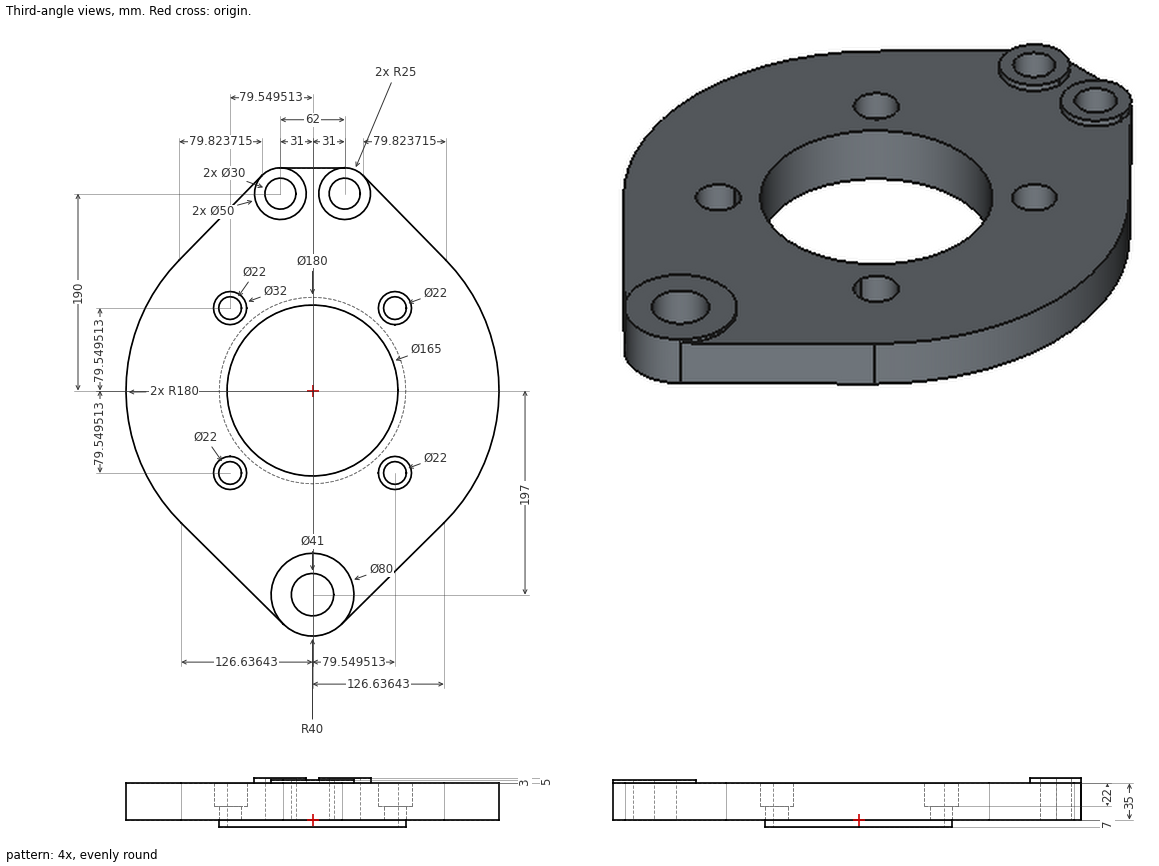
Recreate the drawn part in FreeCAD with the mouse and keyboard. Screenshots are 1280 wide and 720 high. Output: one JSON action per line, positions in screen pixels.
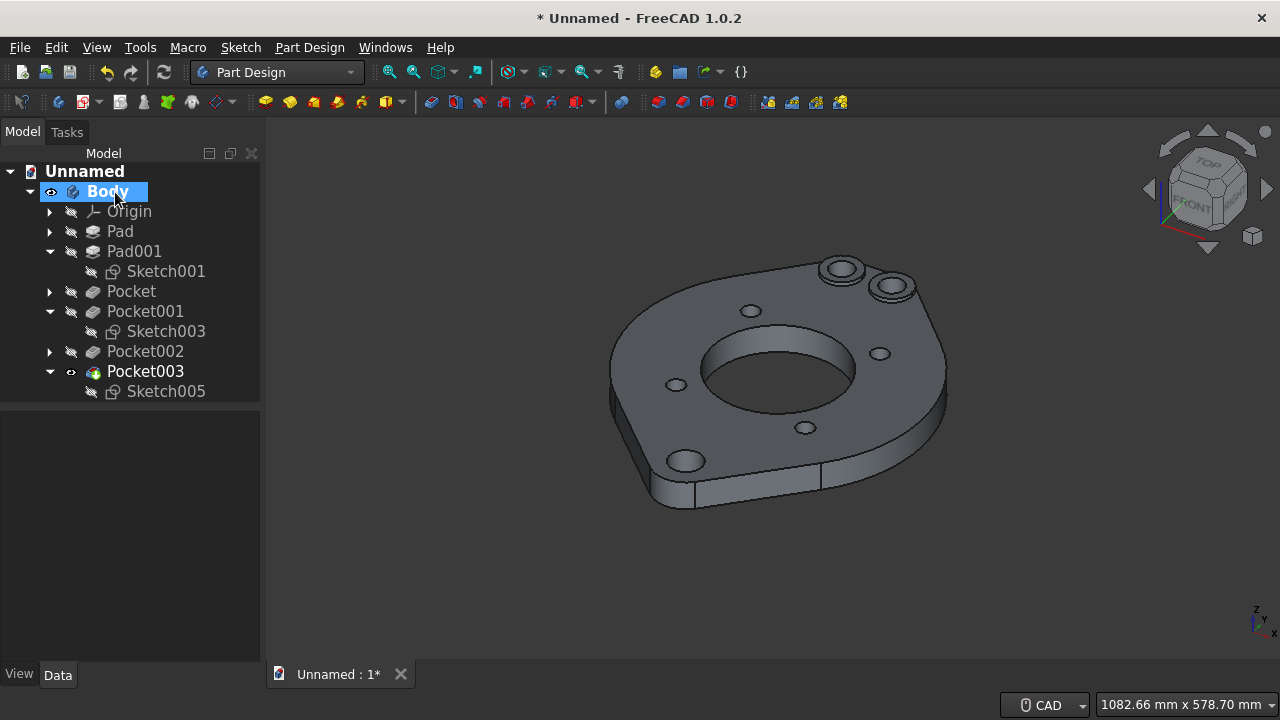
{"action": "left_click", "coordinate": [671, 420]}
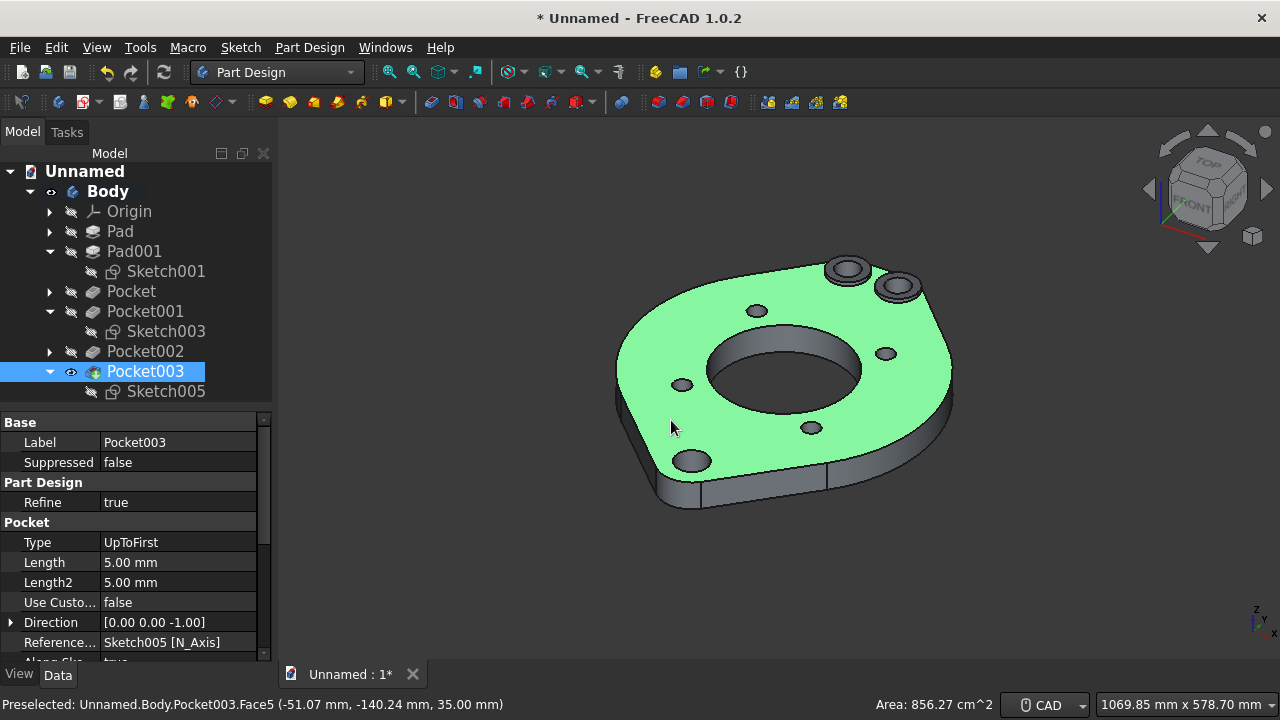
{"action": "left_click", "coordinate": [84, 102]}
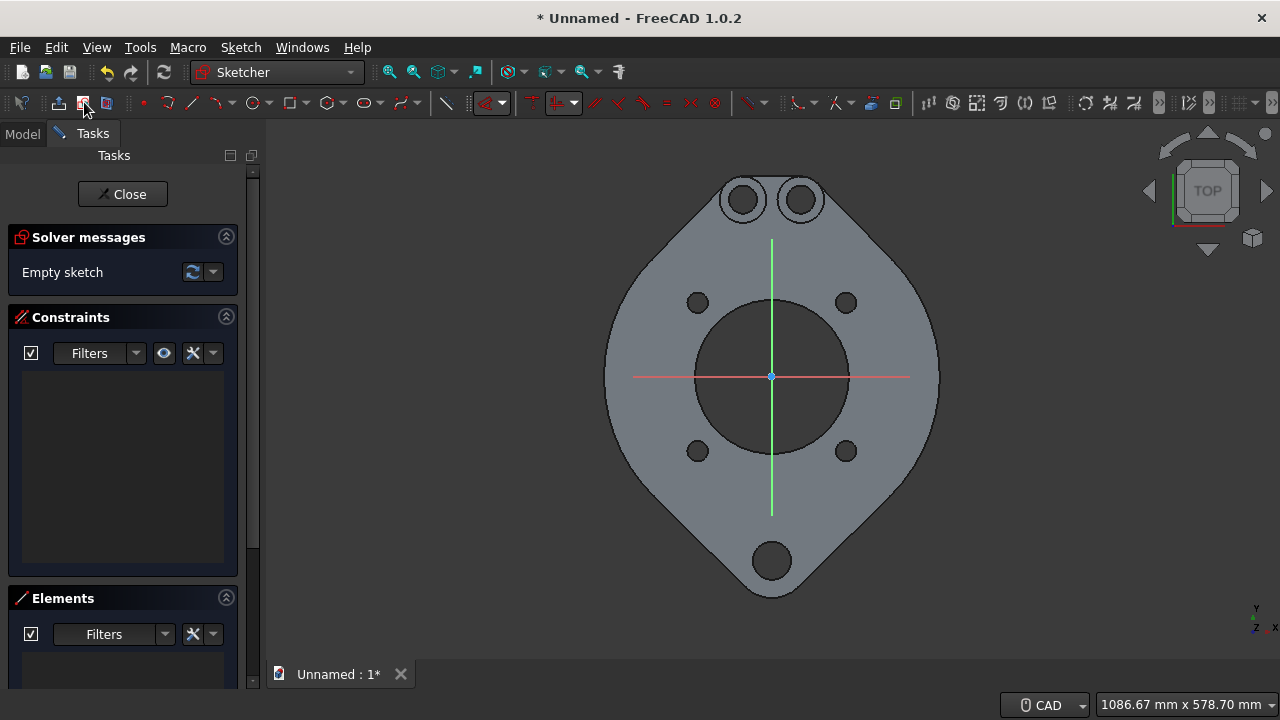
{"action": "left_click", "coordinate": [108, 104]}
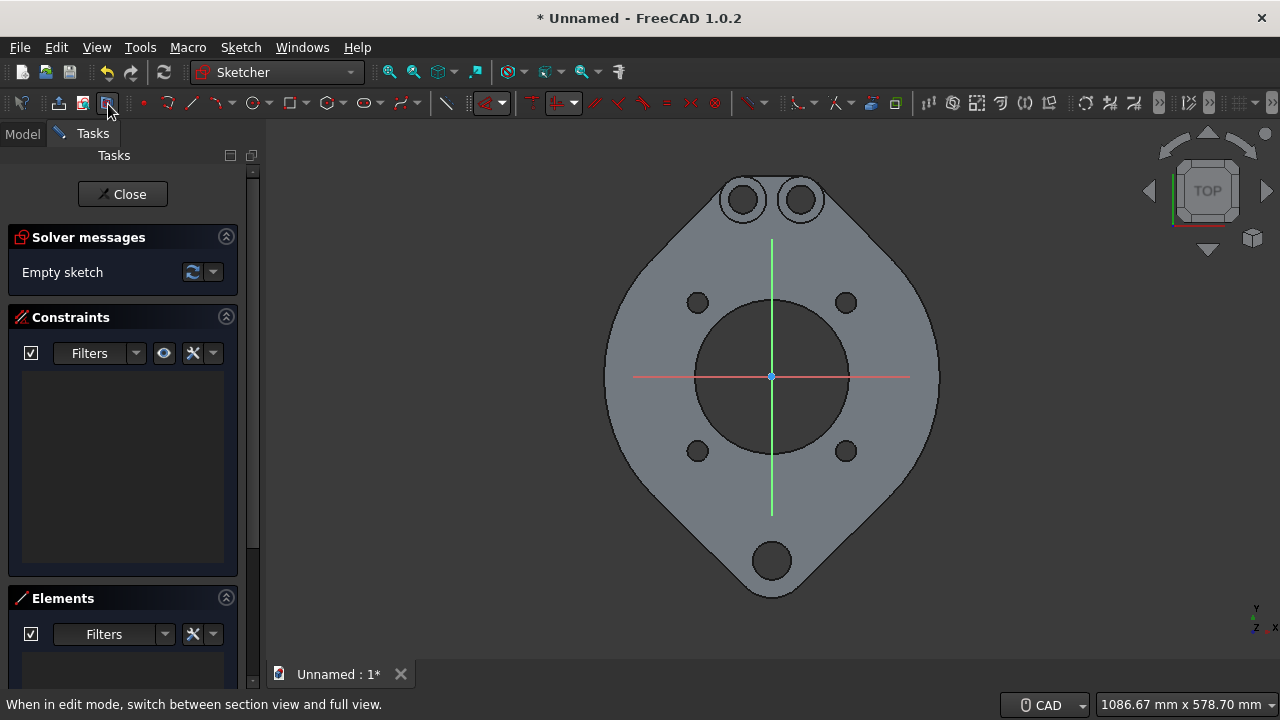
{"action": "scroll", "coordinate": [697, 294], "scroll_direction": "up", "scroll_amount": 12}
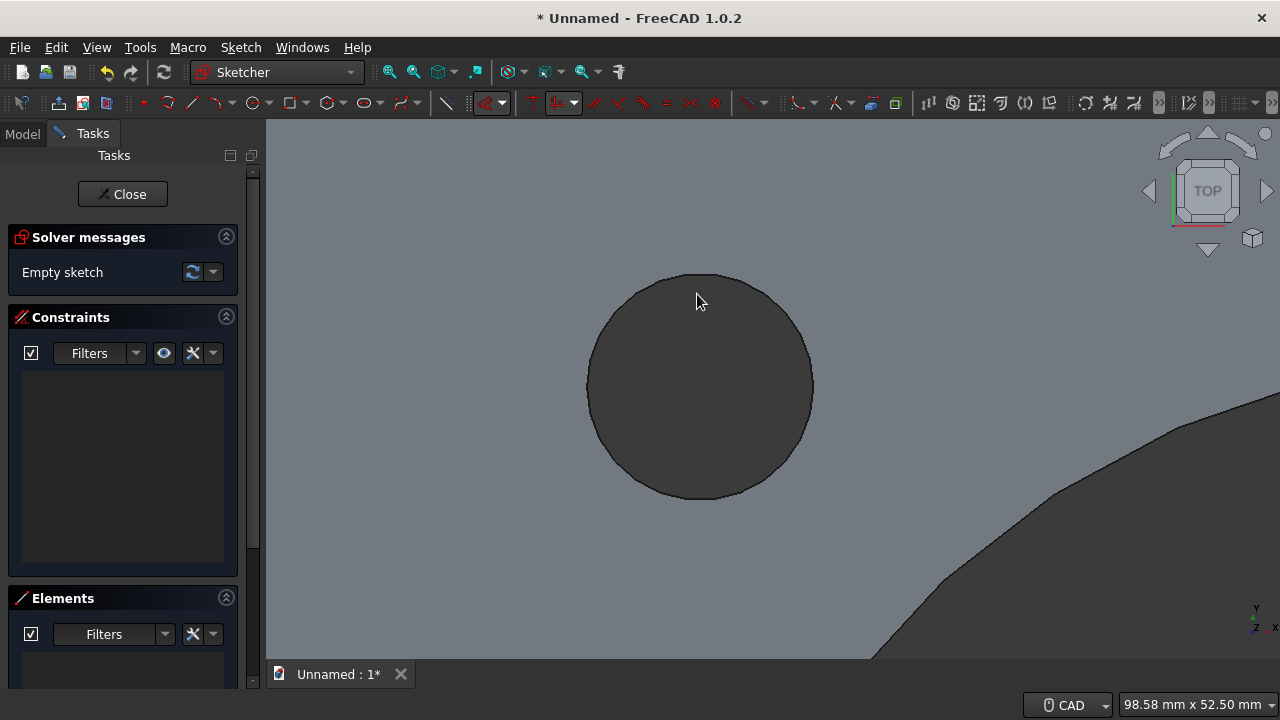
{"action": "key", "text": "g c"}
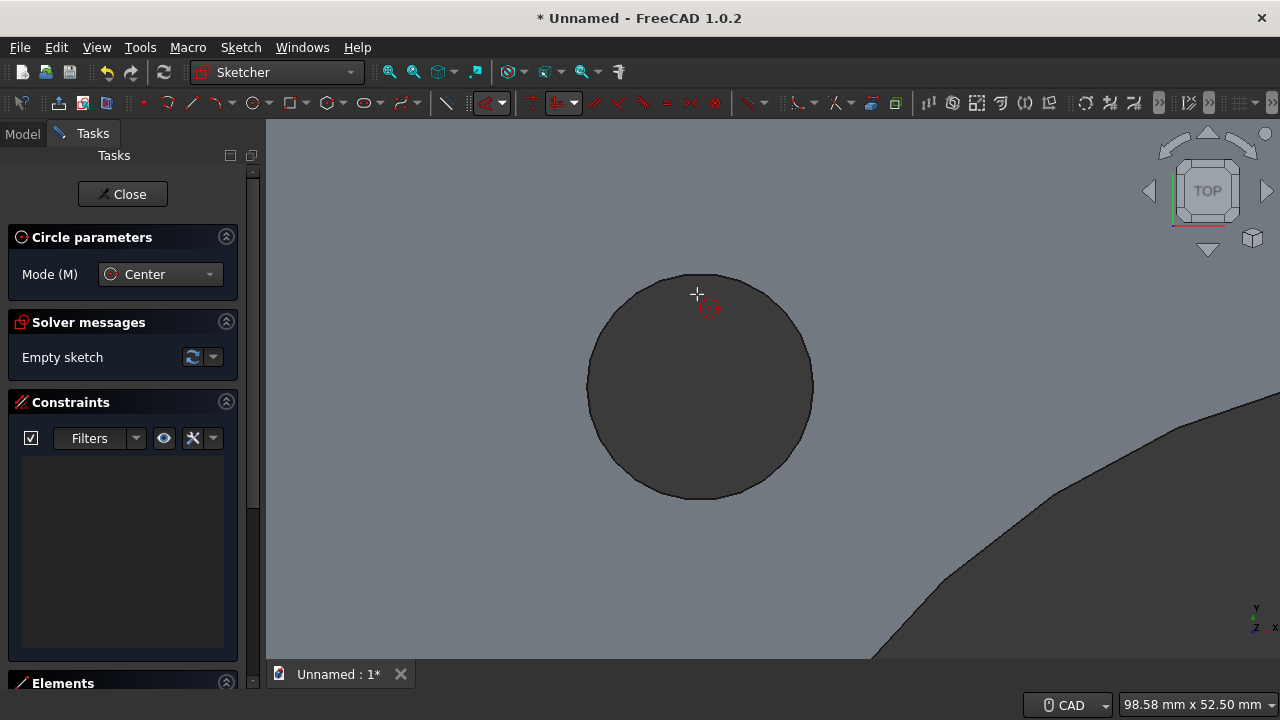
{"action": "left_click", "coordinate": [700, 387]}
{"action": "left_click", "coordinate": [817, 271]}
{"action": "key", "text": "Escape"}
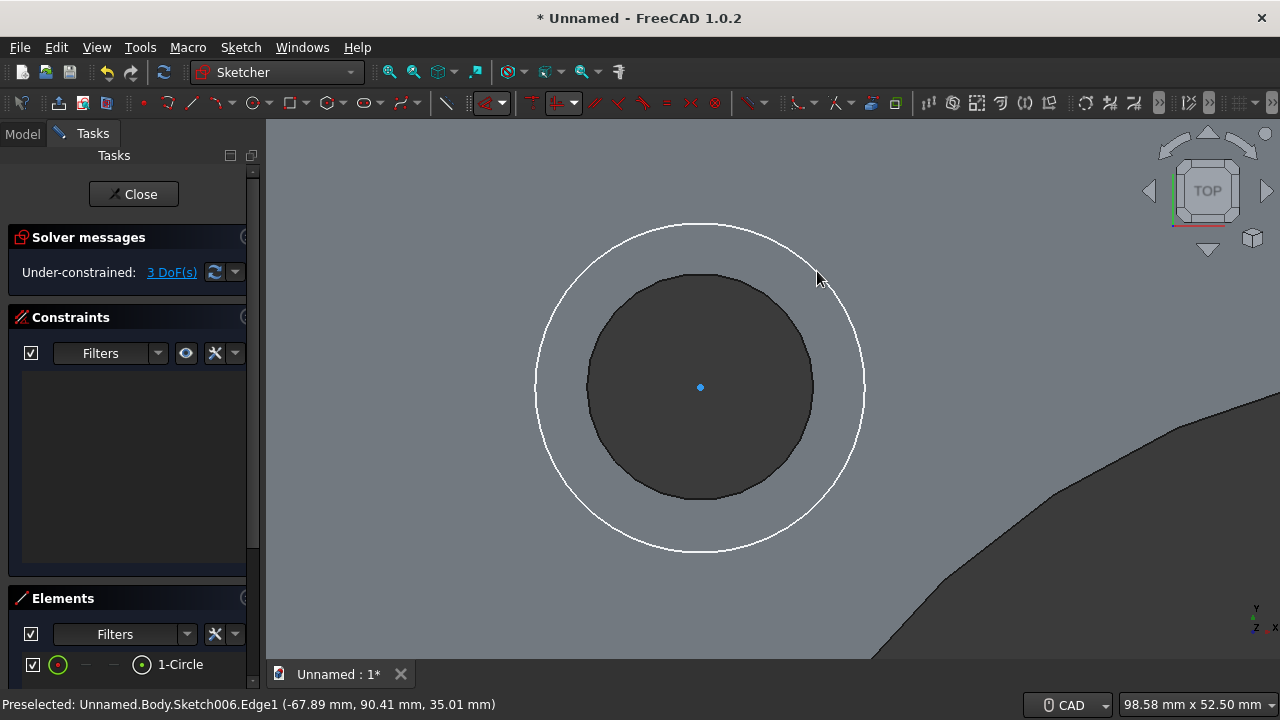
{"action": "left_click", "coordinate": [816, 271]}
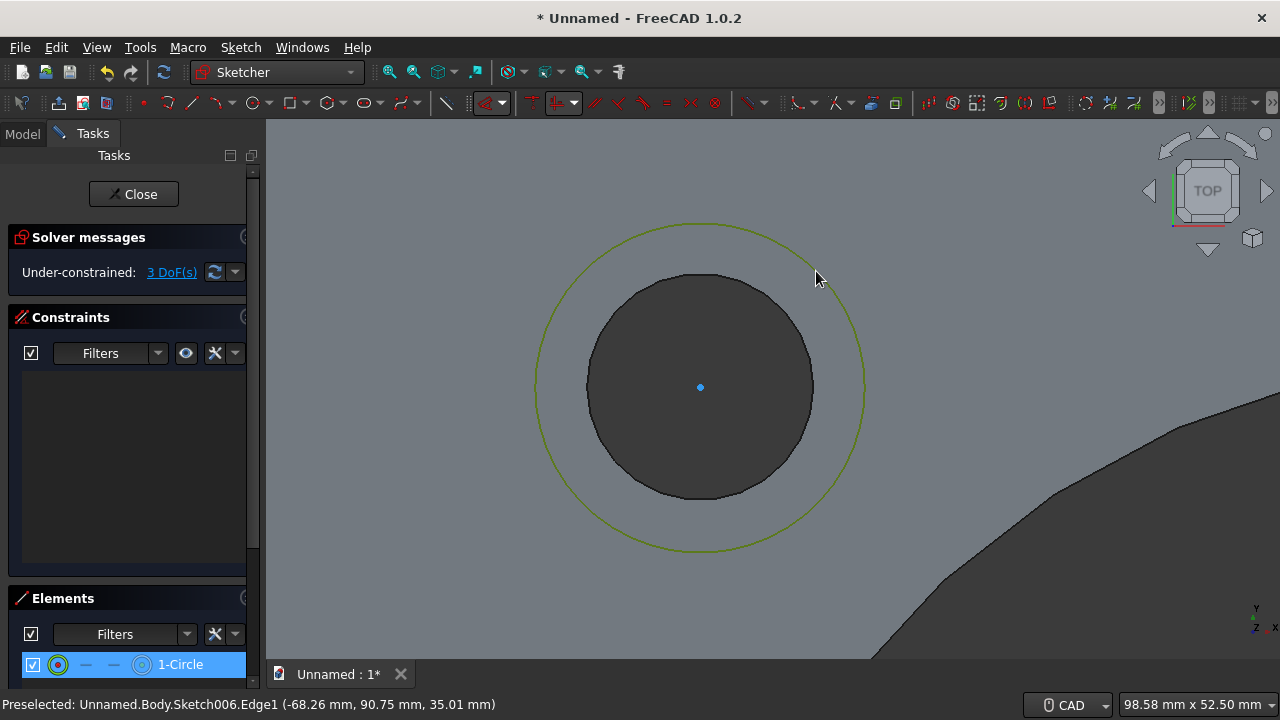
{"action": "left_click", "coordinate": [504, 104]}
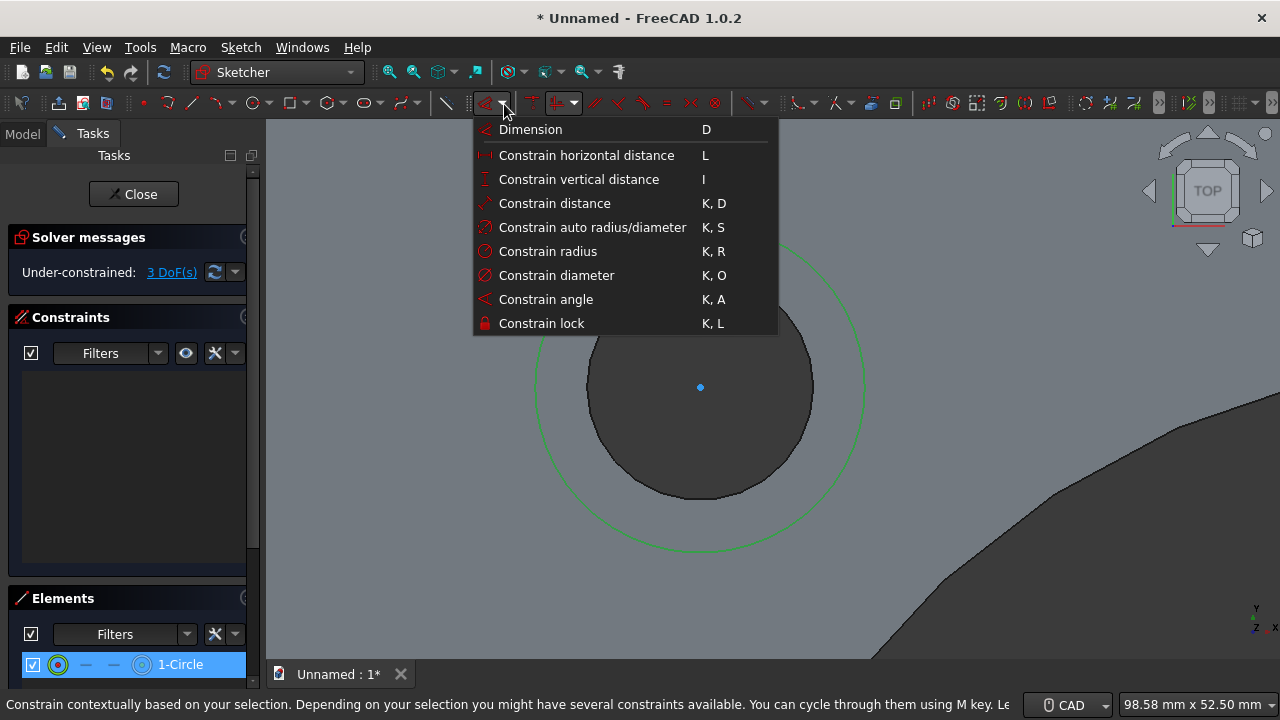
{"action": "left_click", "coordinate": [626, 275]}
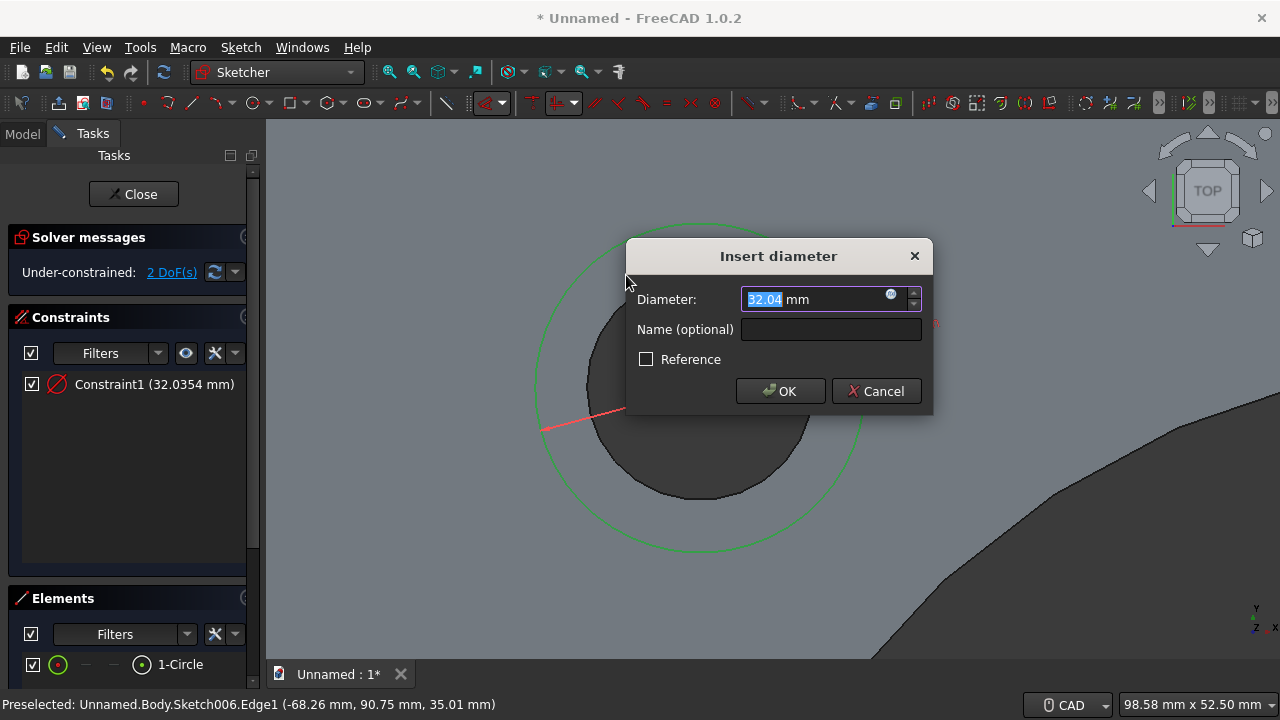
{"action": "type", "text": "32"}
{"action": "key", "text": "Return"}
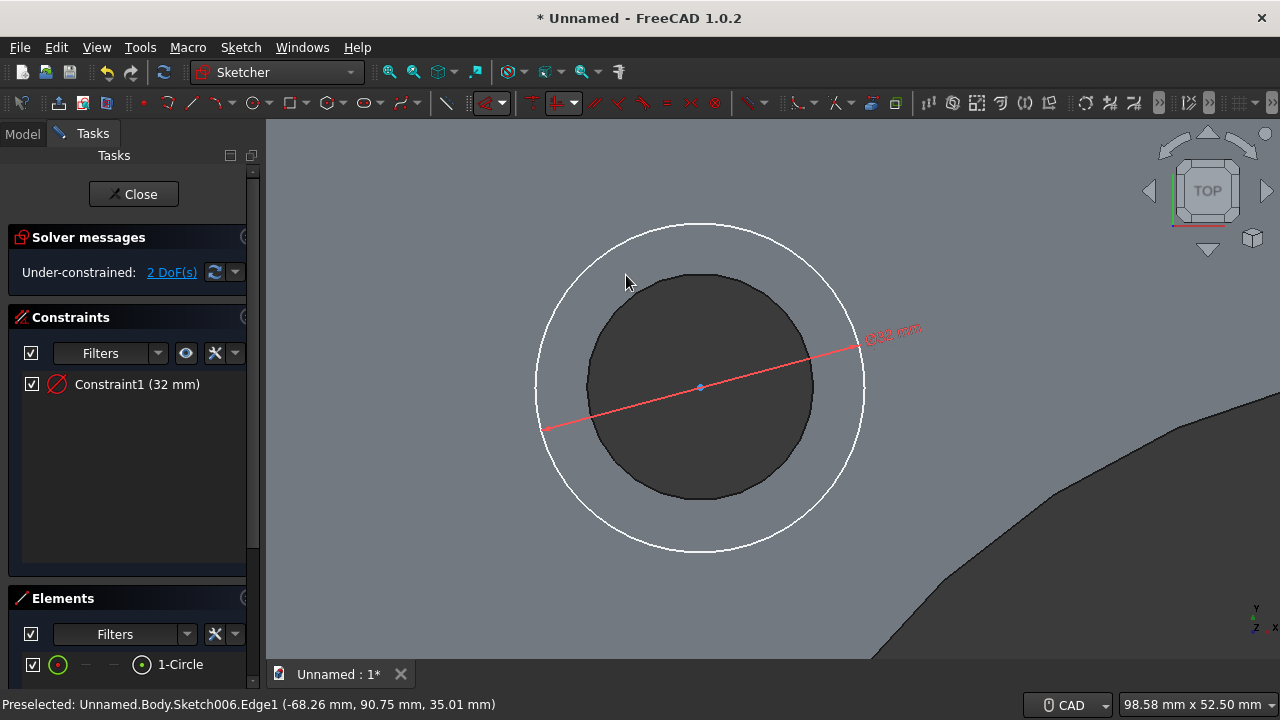
{"action": "left_click", "coordinate": [700, 388]}